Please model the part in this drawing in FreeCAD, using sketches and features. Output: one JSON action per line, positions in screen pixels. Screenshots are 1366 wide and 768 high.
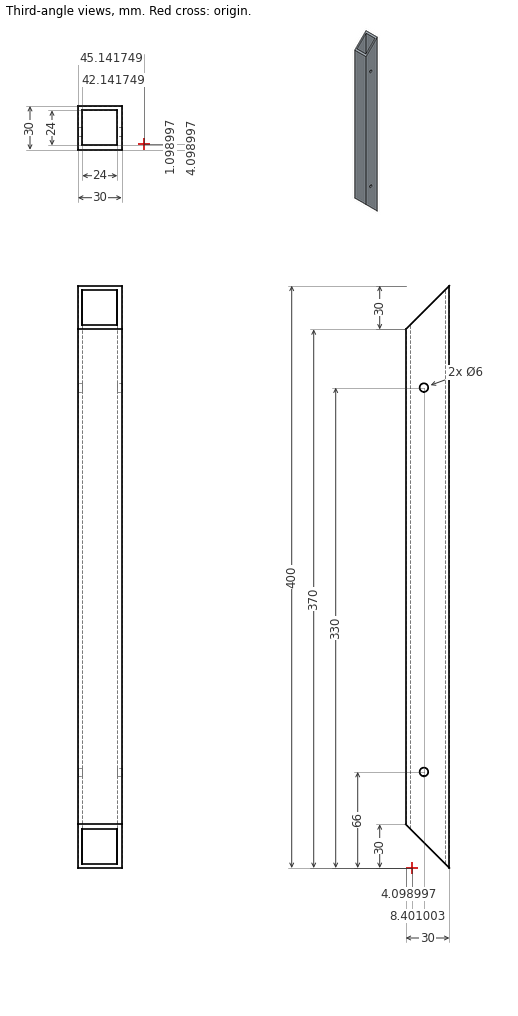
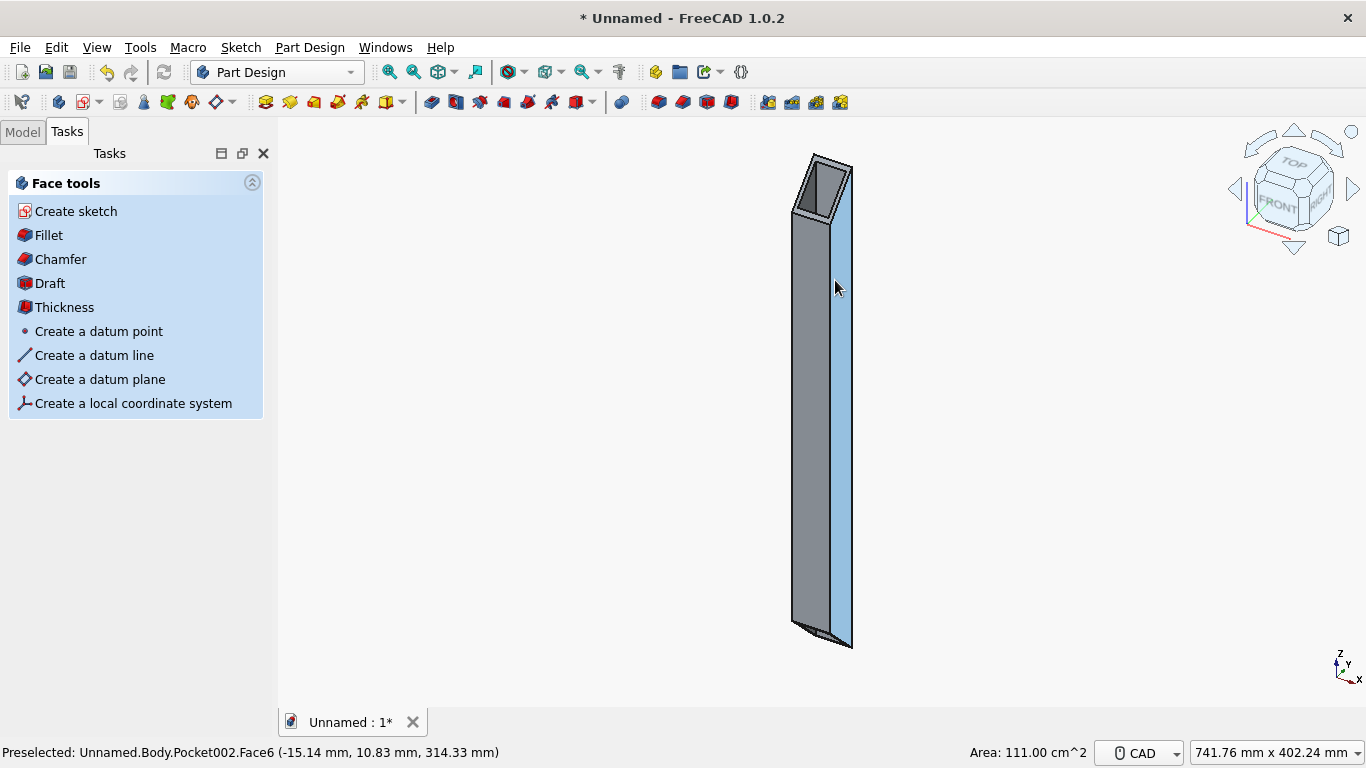
{"action": "left_click", "coordinate": [84, 102]}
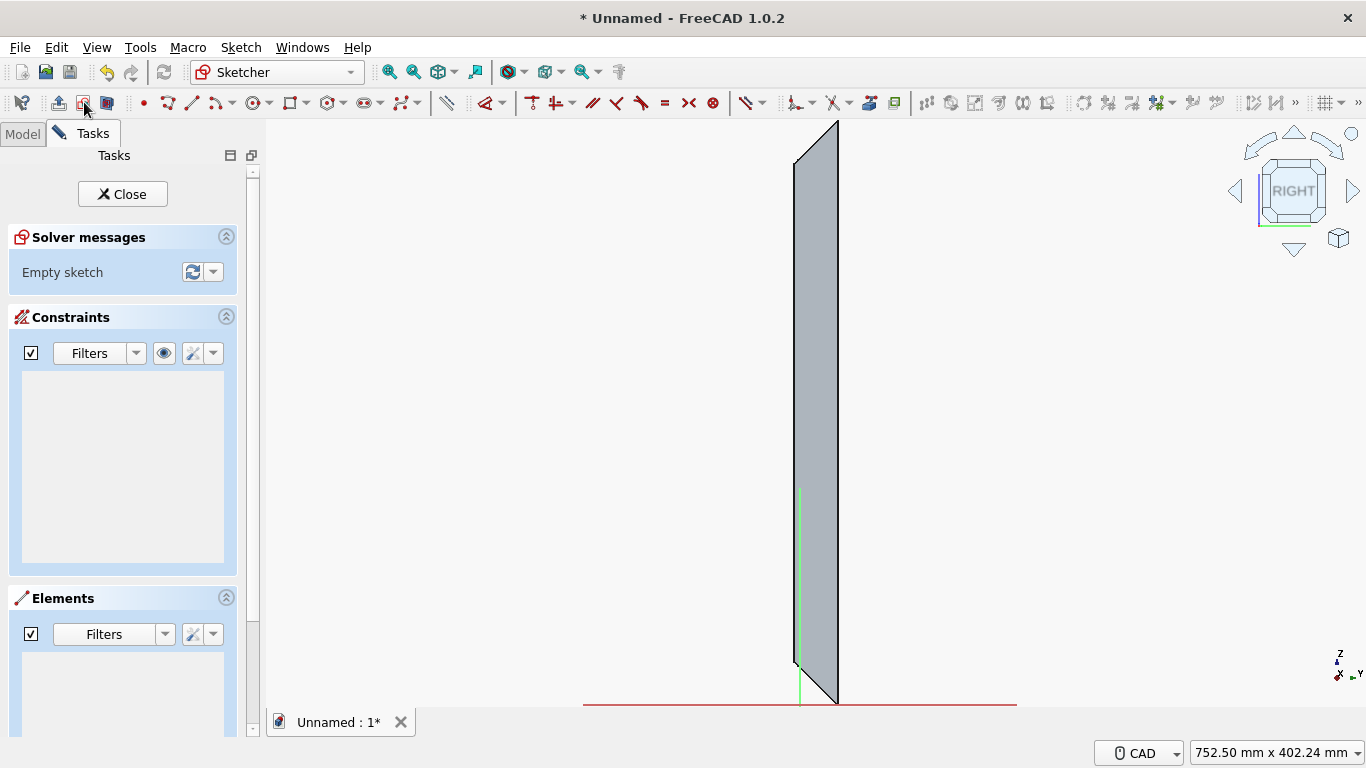
{"action": "scroll", "coordinate": [472, 192], "scroll_direction": "down", "scroll_amount": 1}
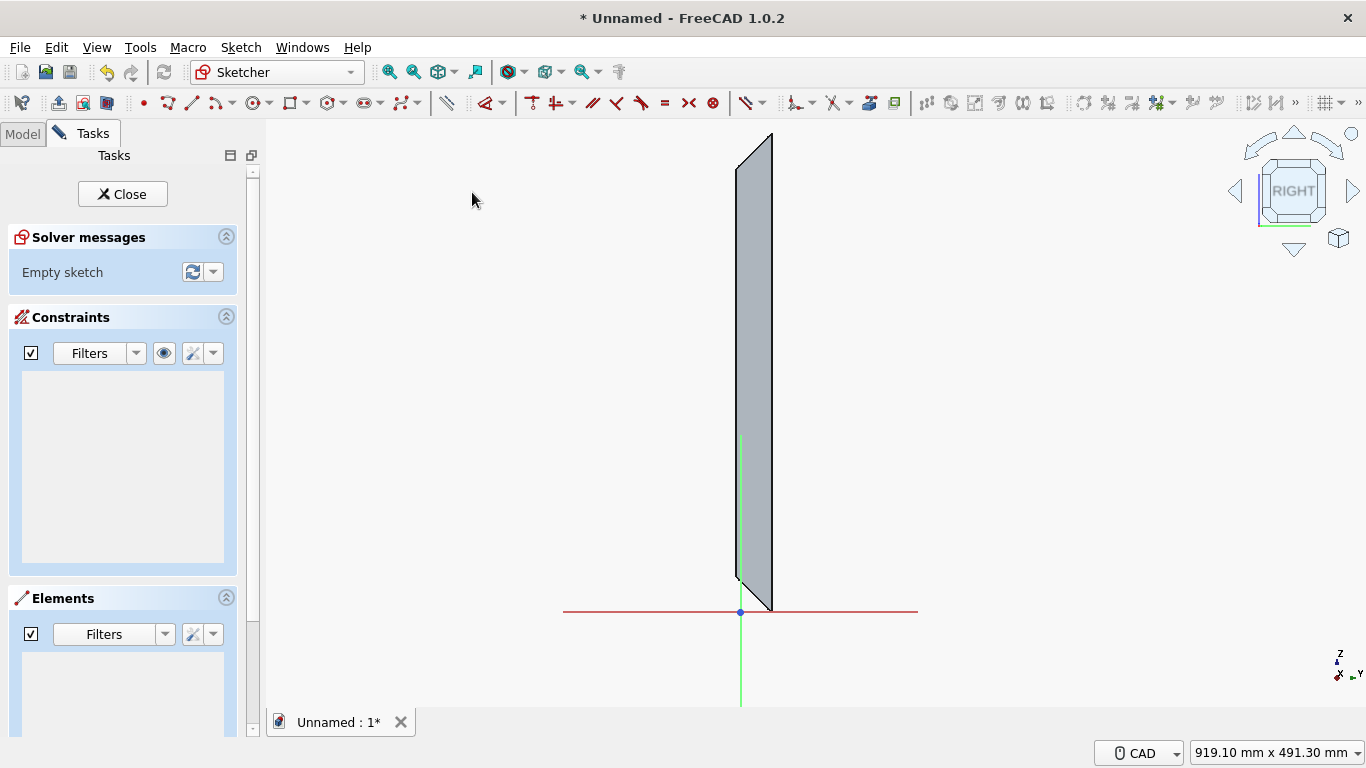
{"action": "left_click", "coordinate": [254, 104]}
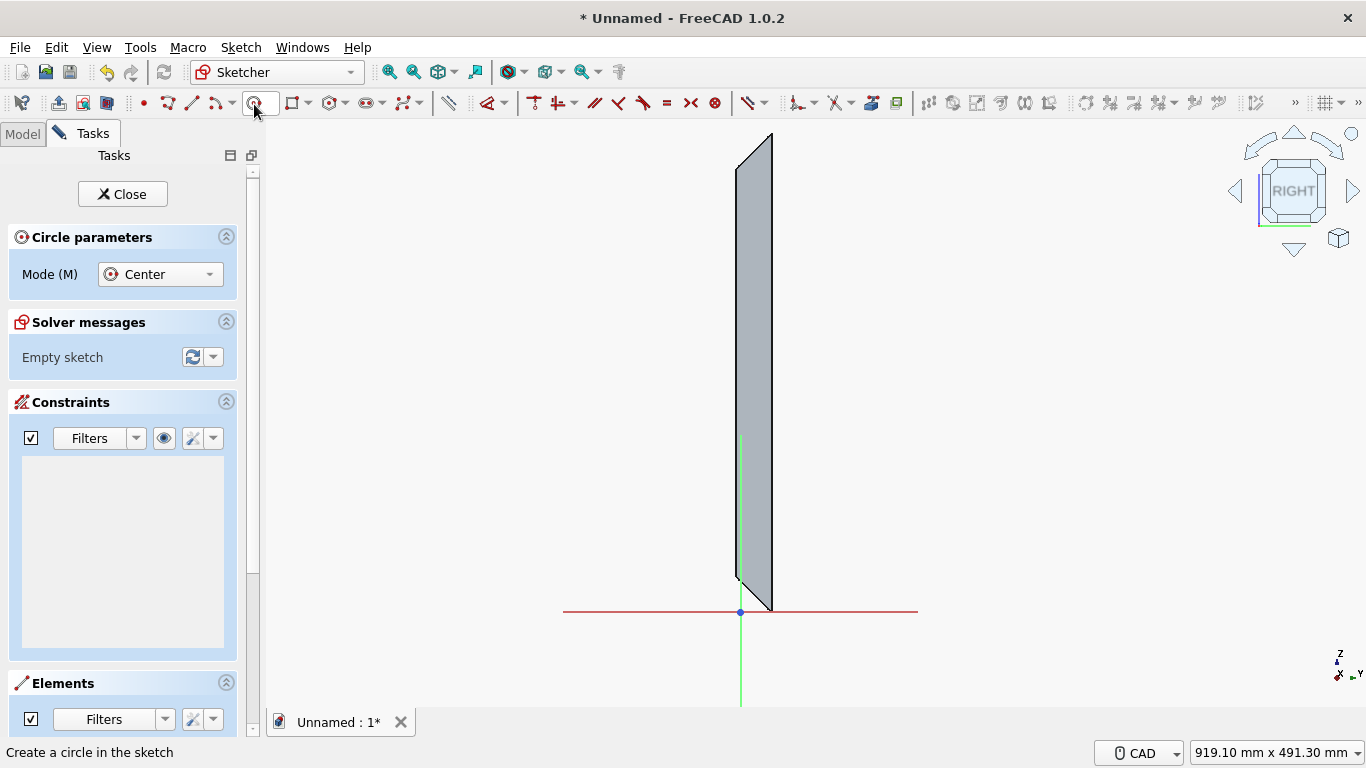
{"action": "scroll", "coordinate": [751, 217], "scroll_direction": "up", "scroll_amount": 10}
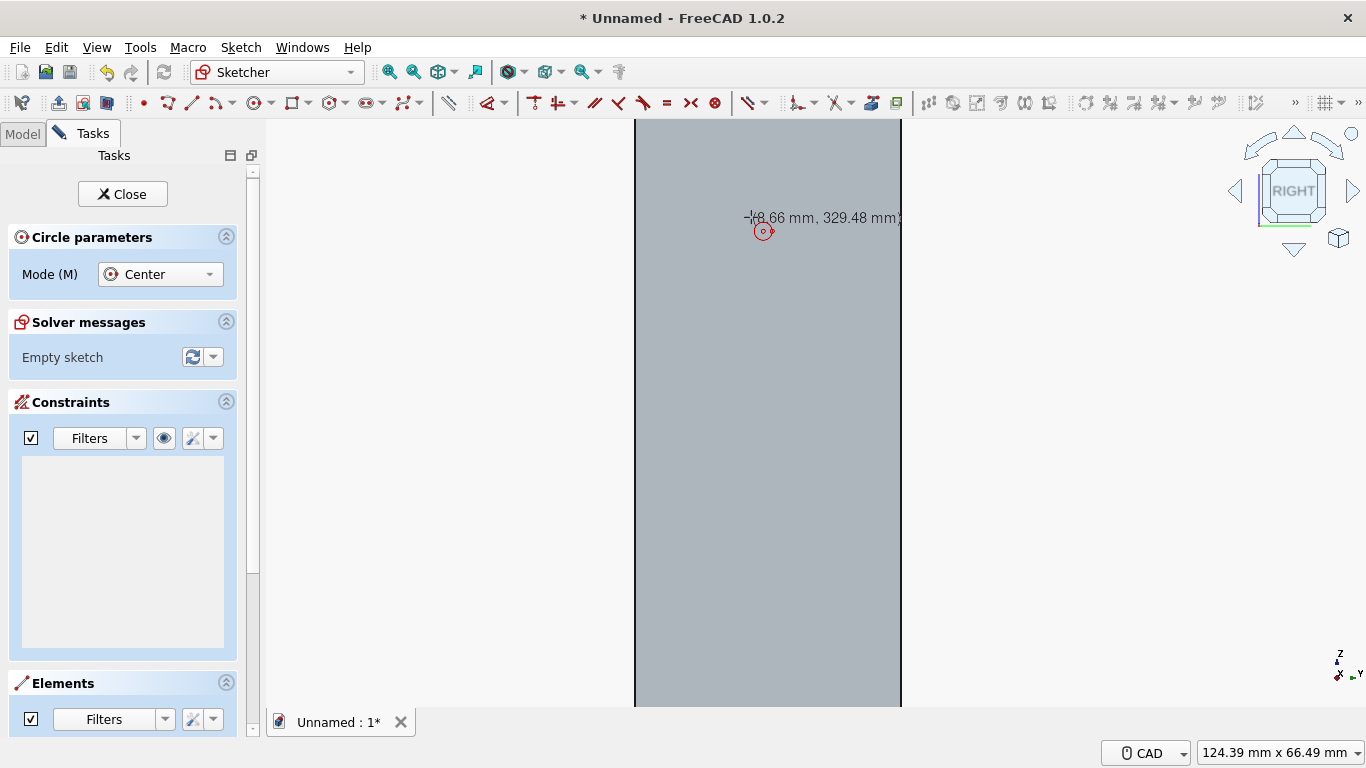
{"action": "scroll", "coordinate": [751, 217], "scroll_direction": "down", "scroll_amount": 10}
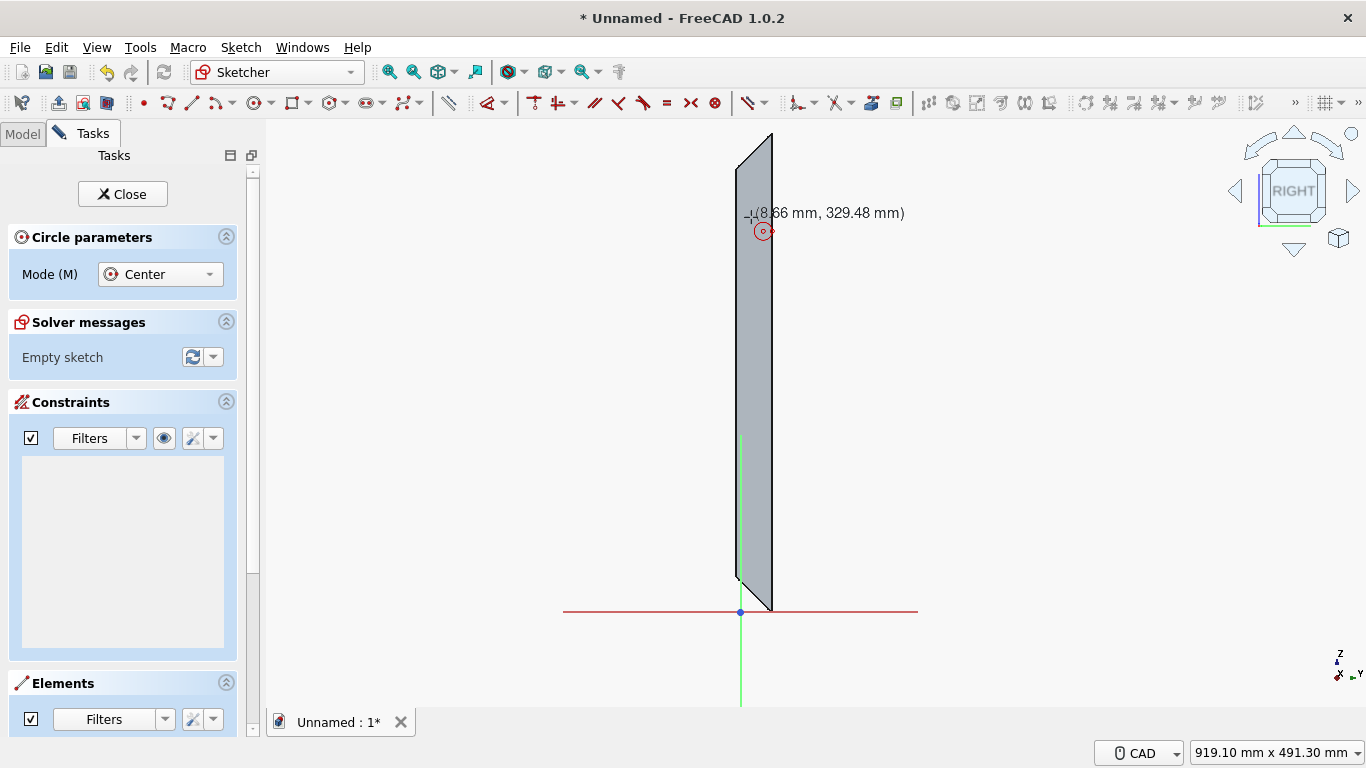
{"action": "scroll", "coordinate": [751, 217], "scroll_direction": "up", "scroll_amount": 3}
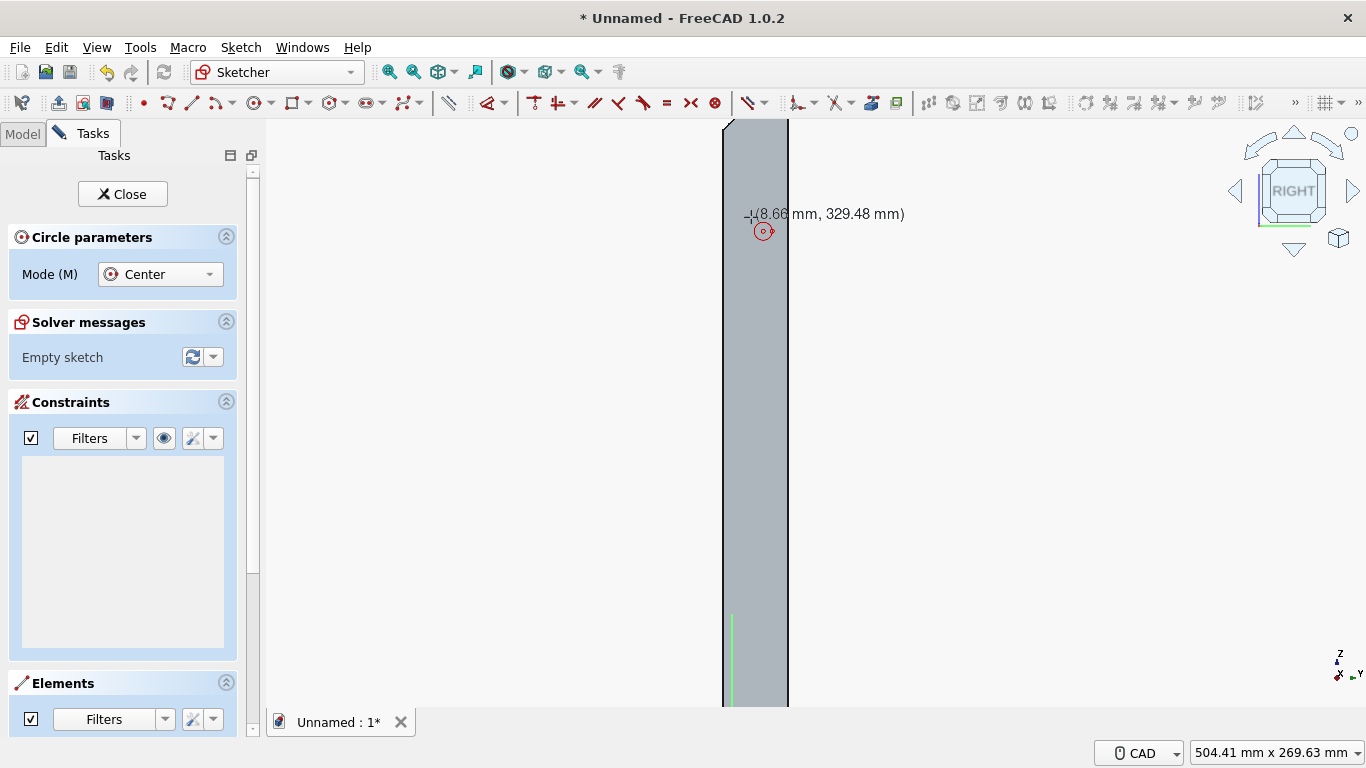
{"action": "left_click", "coordinate": [750, 218]}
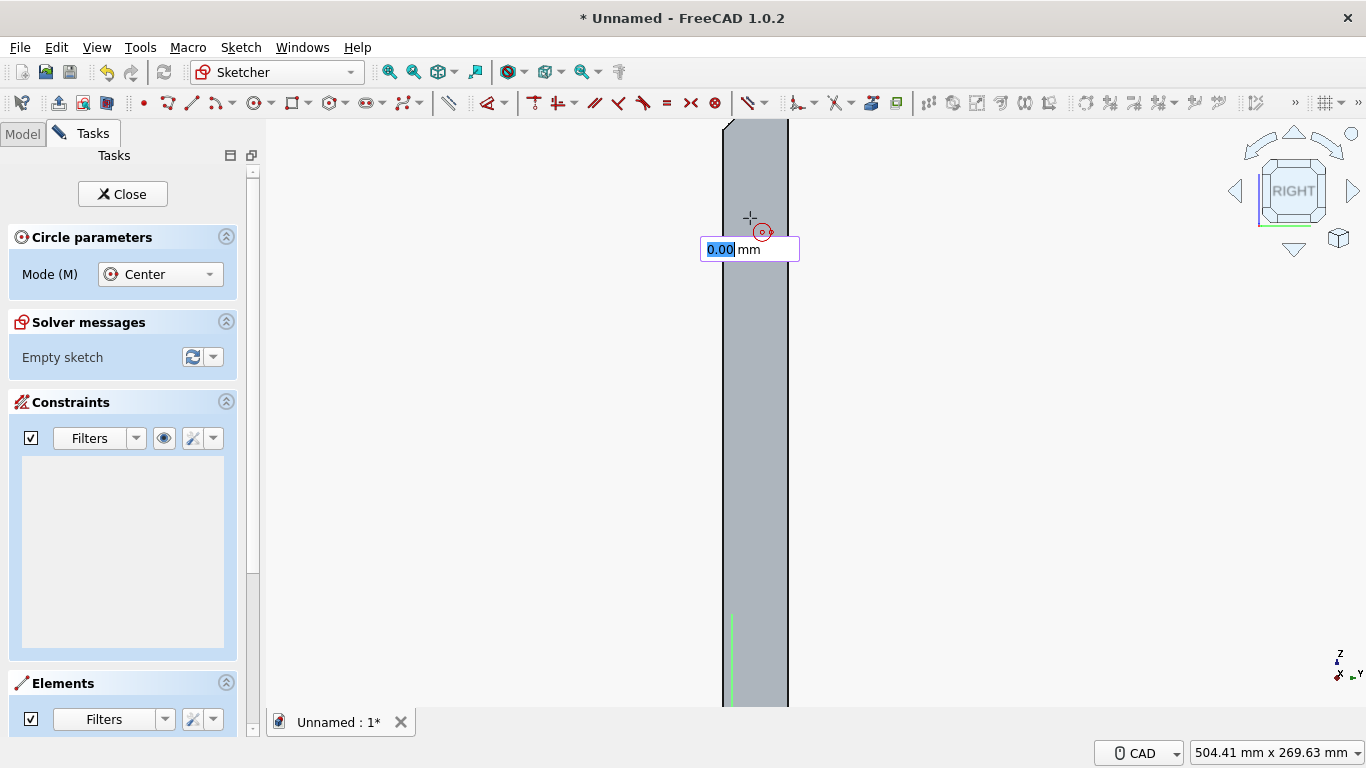
{"action": "scroll", "coordinate": [755, 213], "scroll_direction": "up", "scroll_amount": 5}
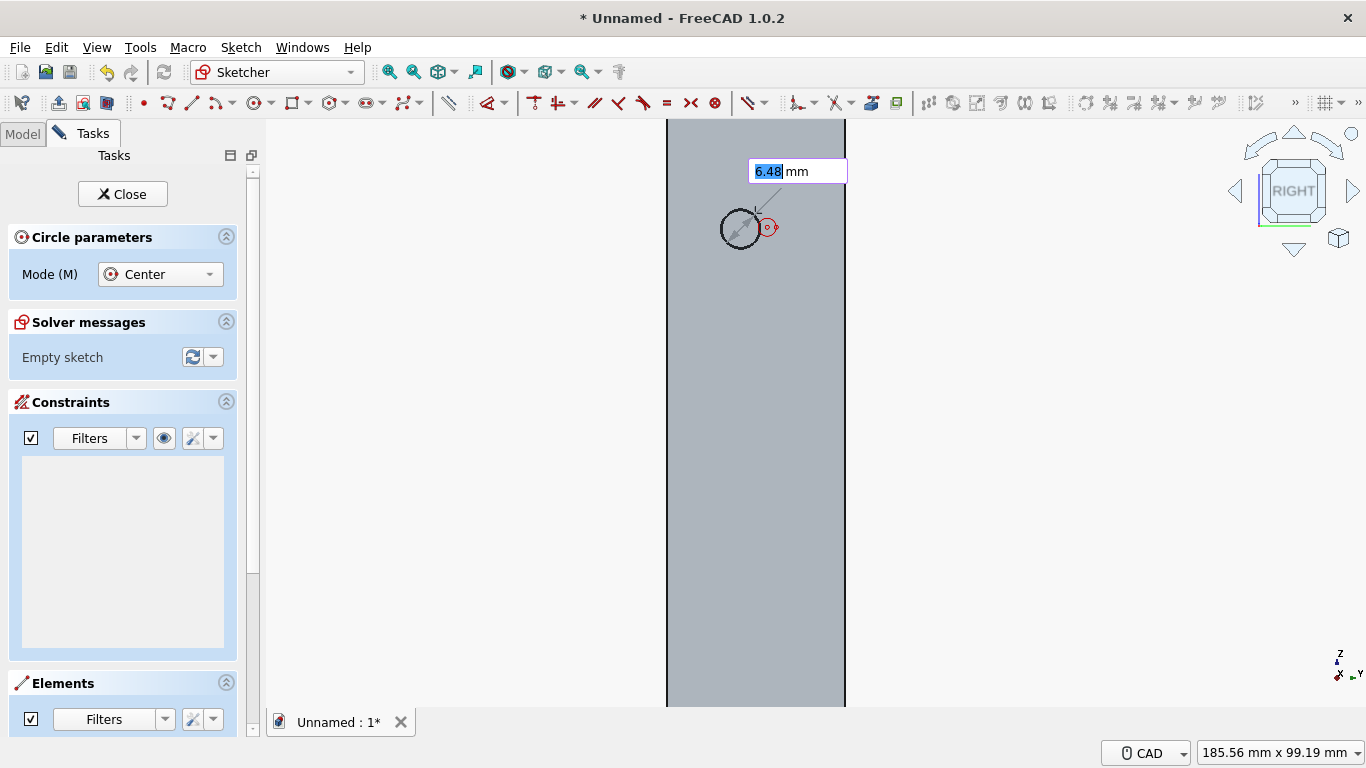
{"action": "left_click", "coordinate": [753, 213]}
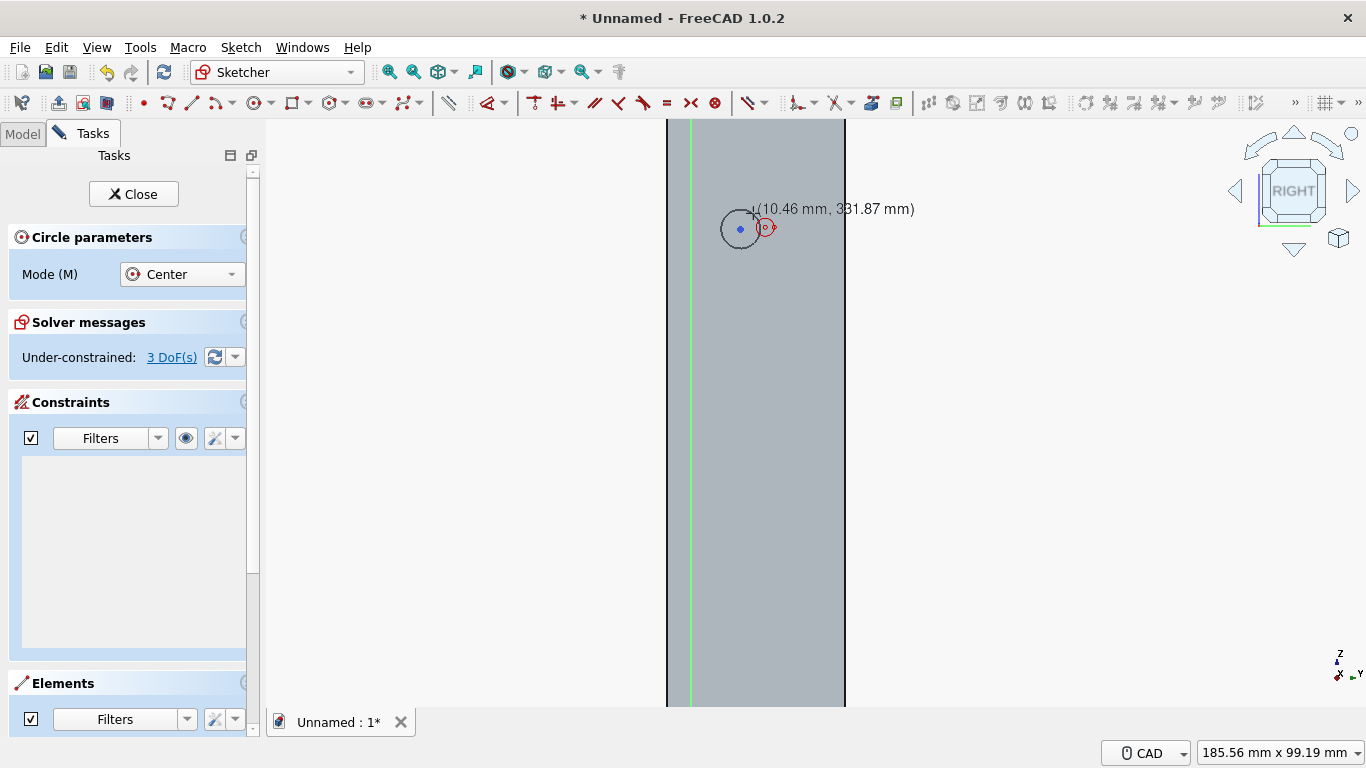
{"action": "scroll", "coordinate": [753, 215], "scroll_direction": "down", "scroll_amount": 8}